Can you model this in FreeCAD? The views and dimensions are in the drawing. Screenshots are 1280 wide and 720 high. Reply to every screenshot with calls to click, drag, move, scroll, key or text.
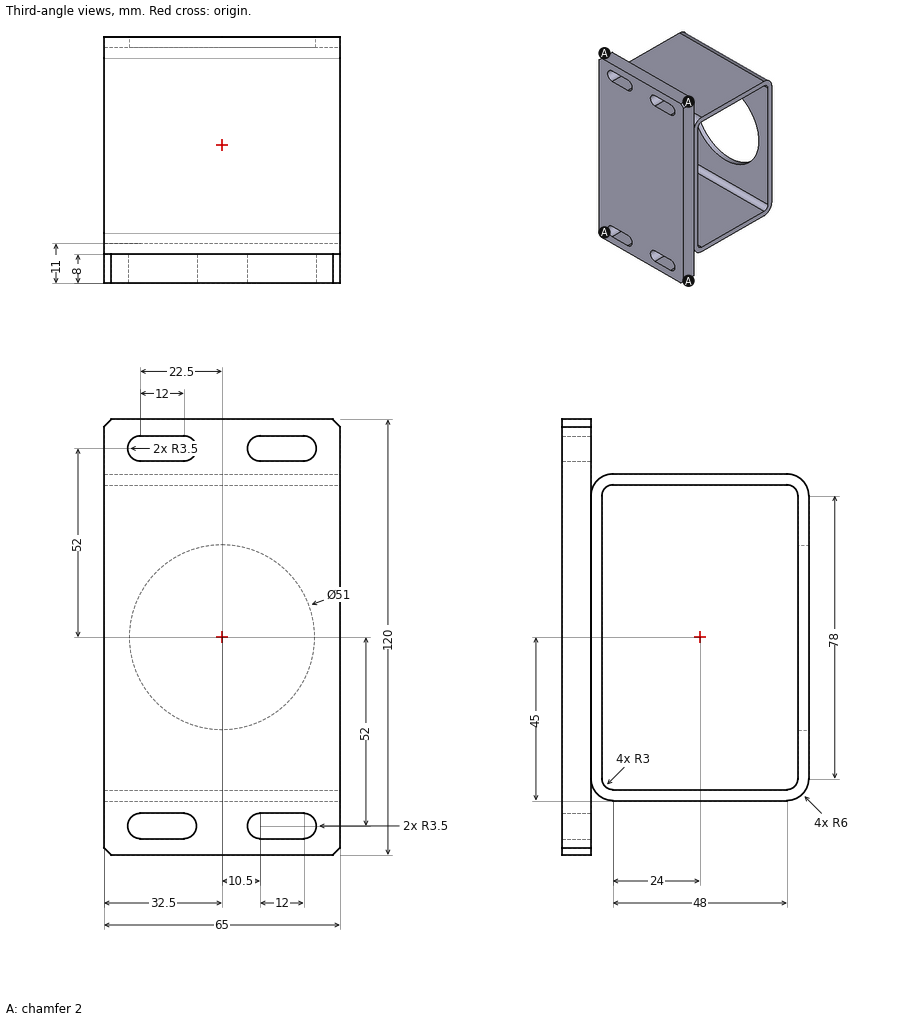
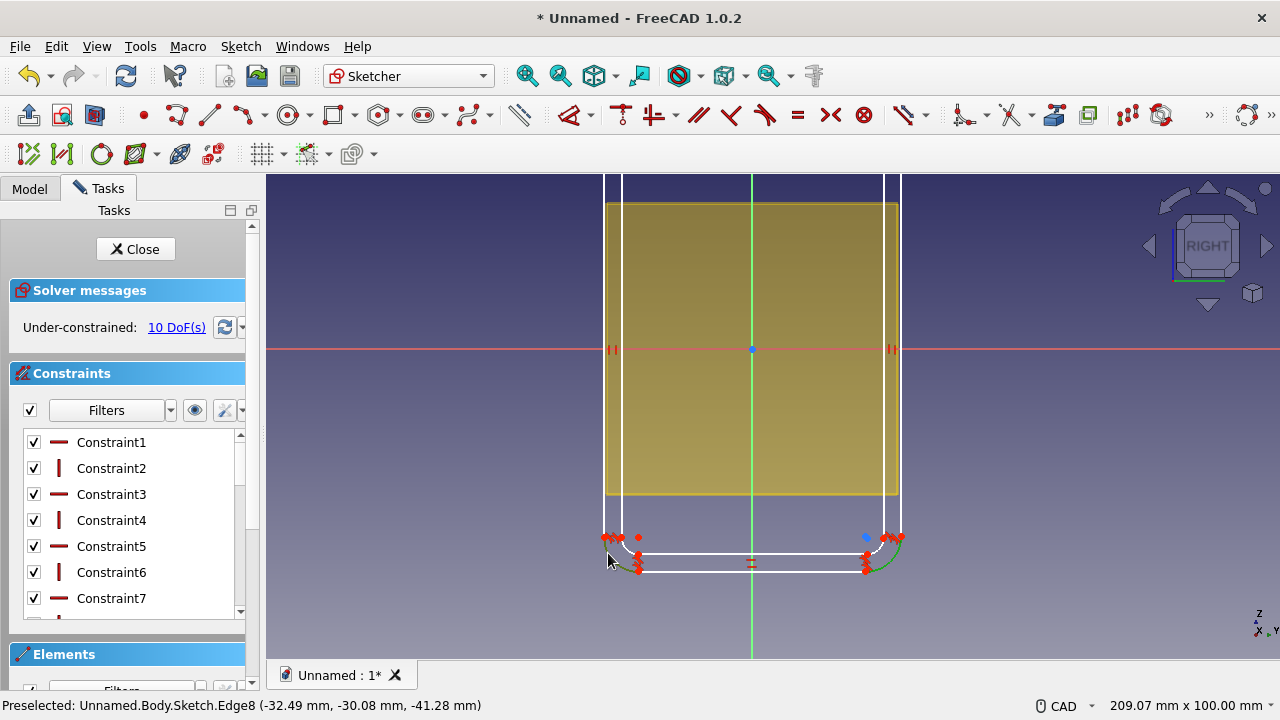
click(798, 116)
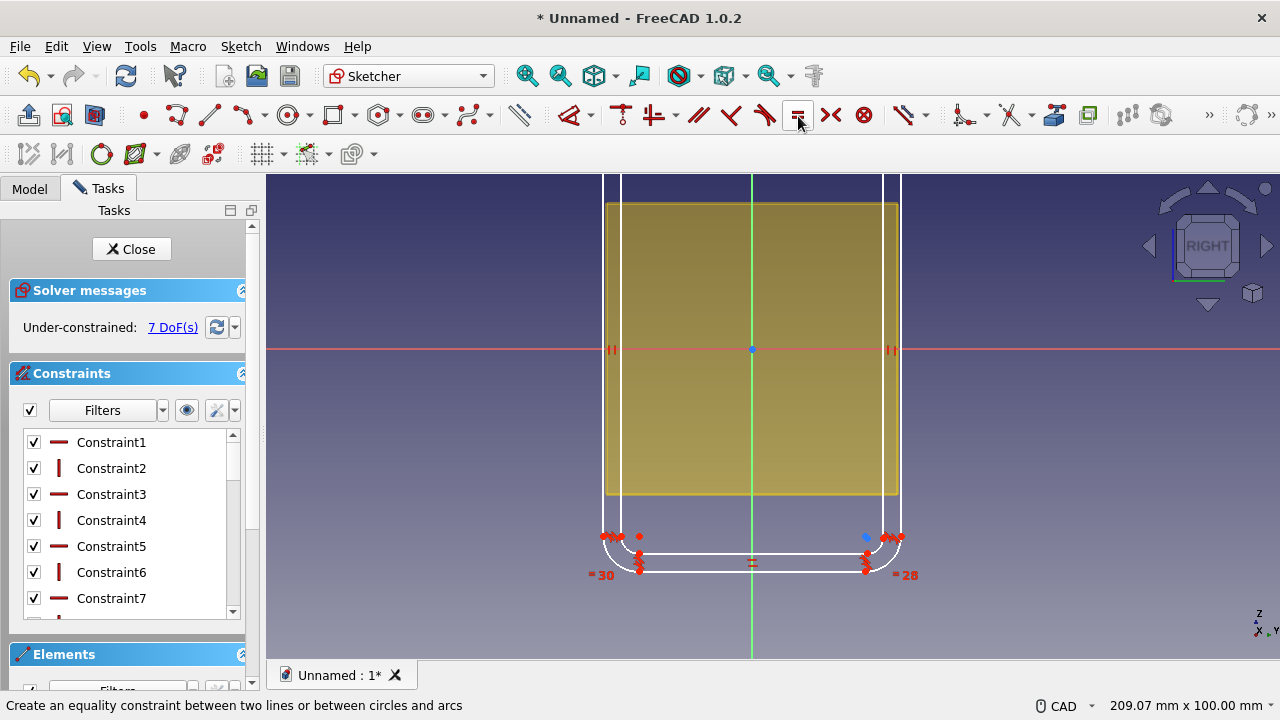
click(626, 549)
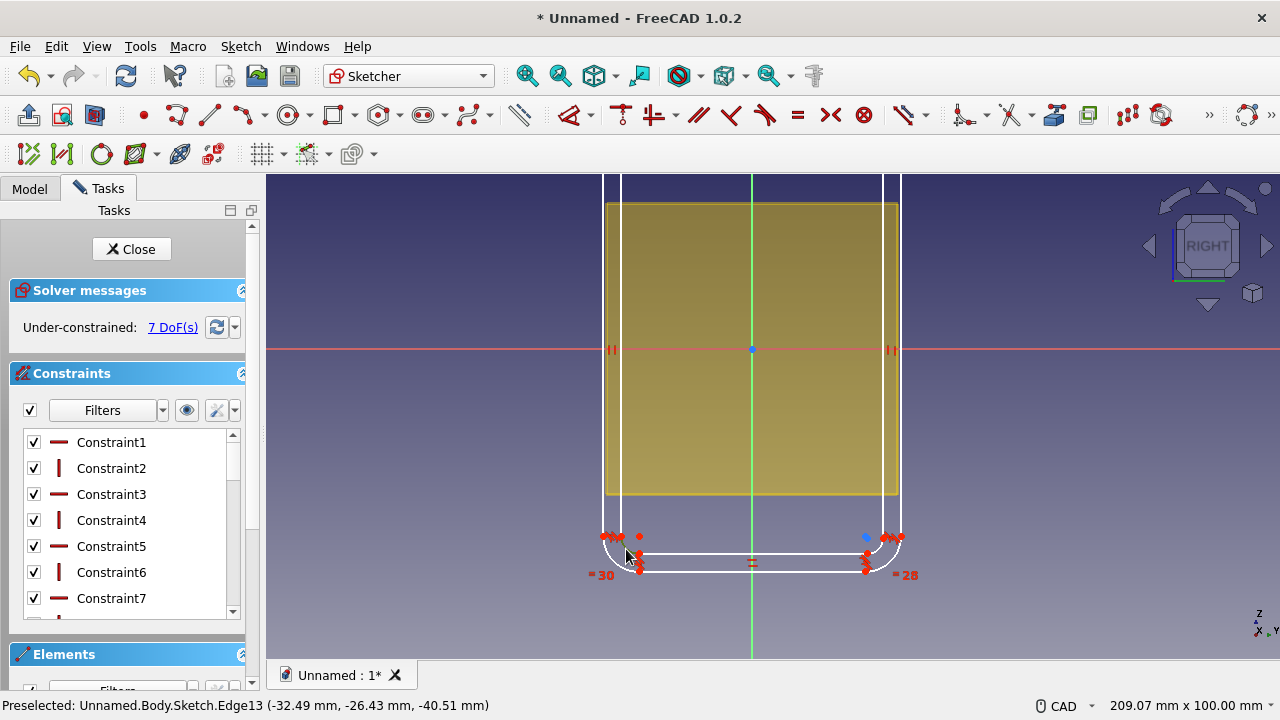
click(878, 549)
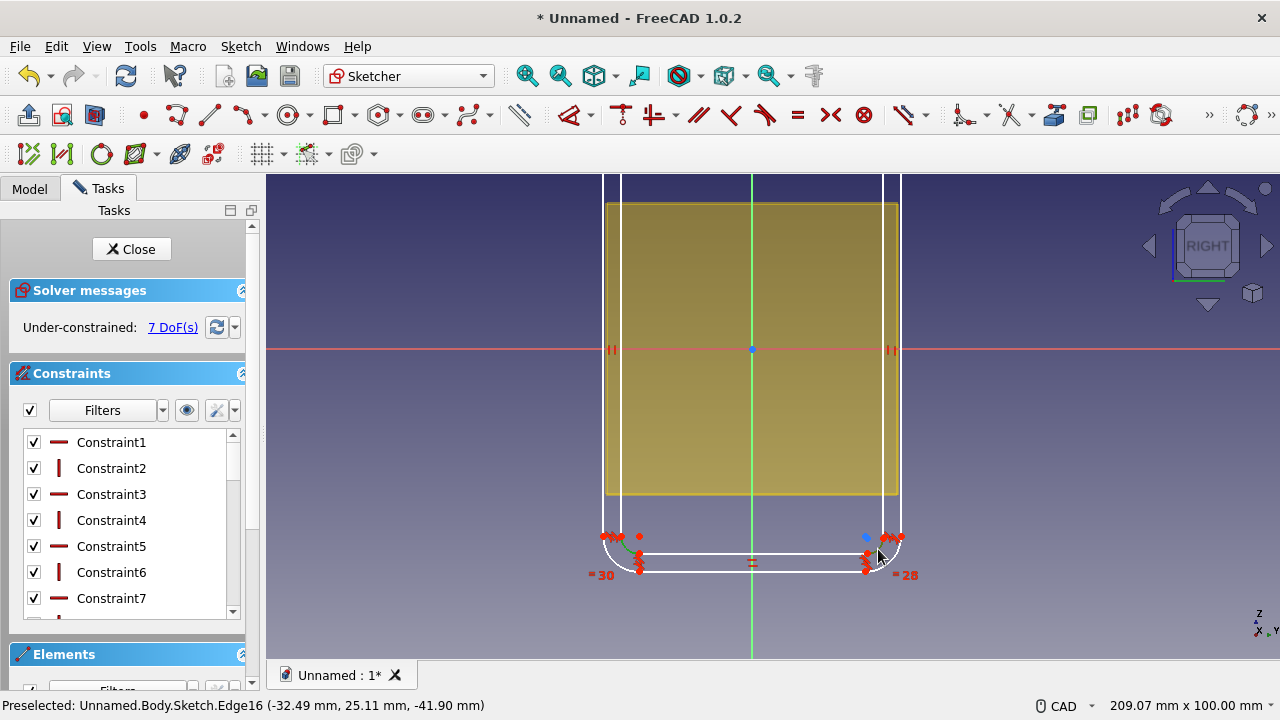
click(798, 116)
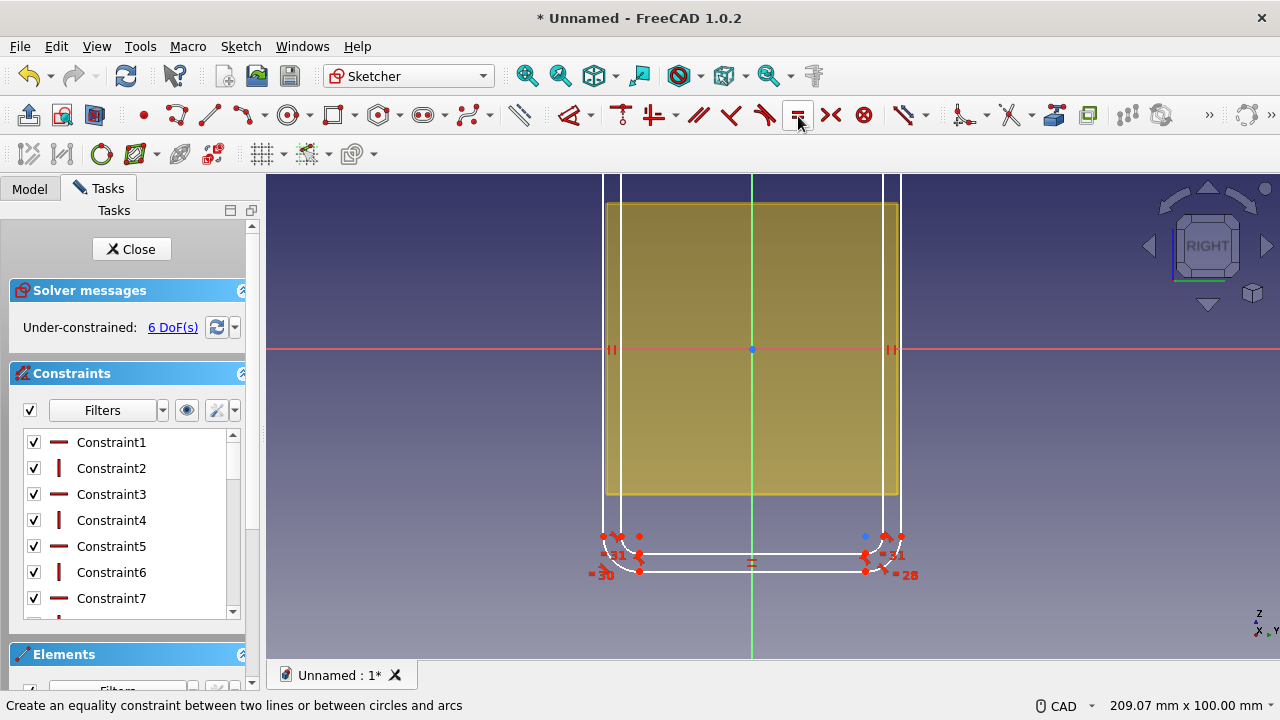
click(568, 116)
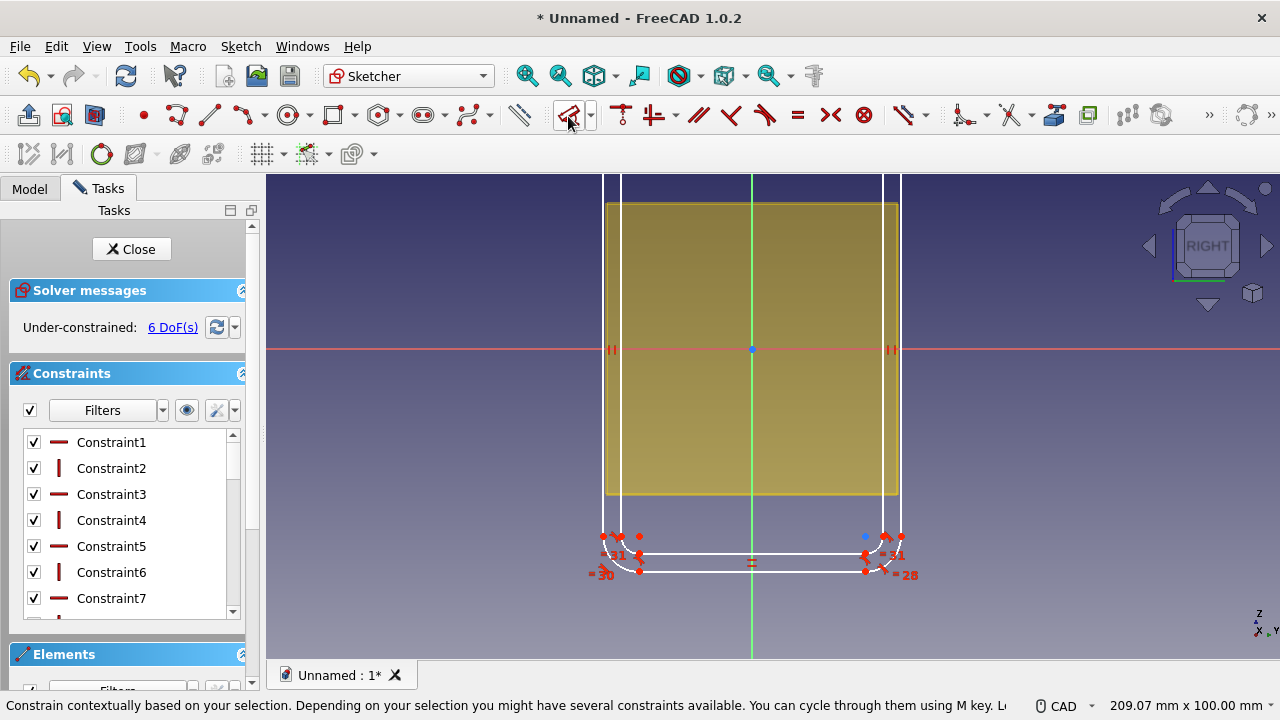
scroll(882, 568, up, 2)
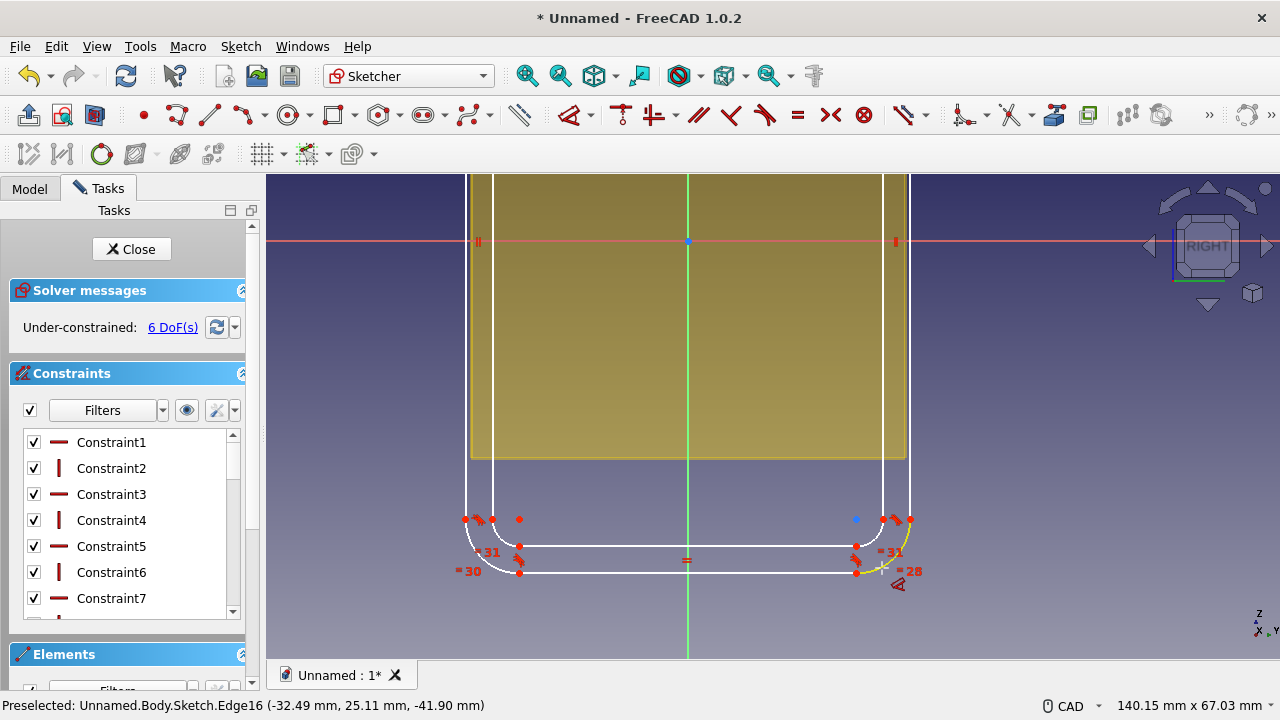
click(881, 568)
click(895, 597)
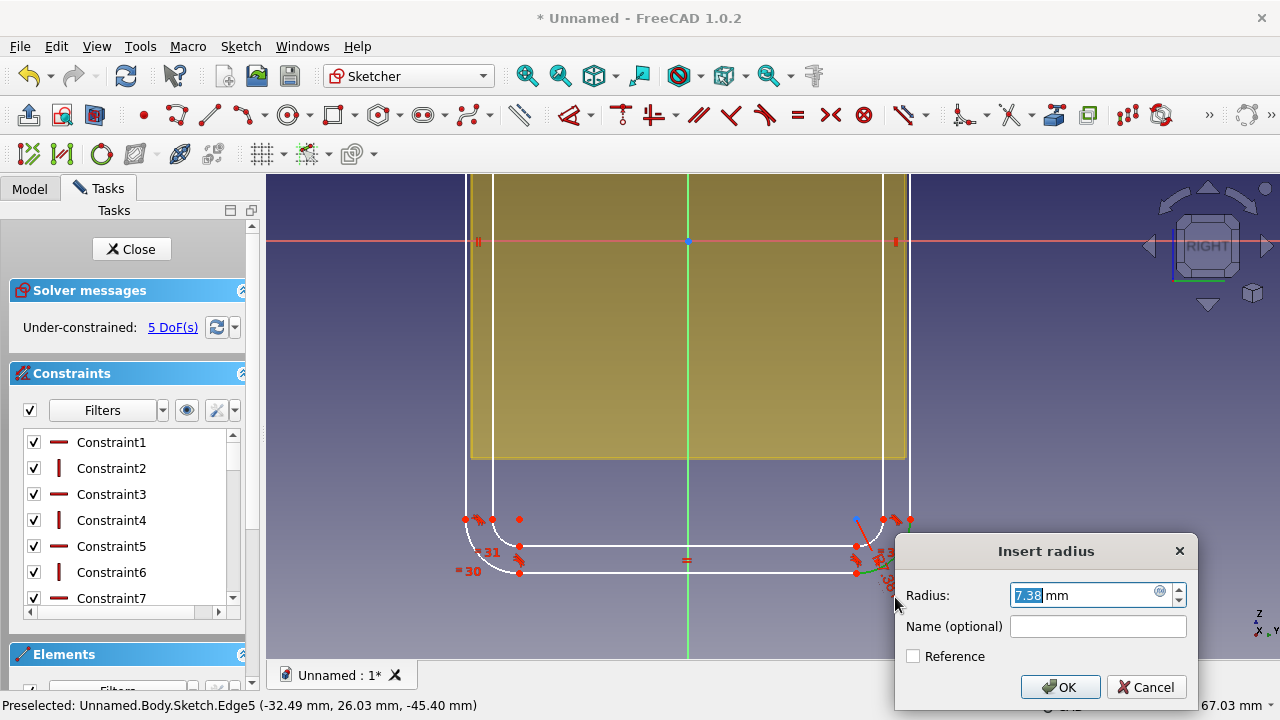
text(6)
key(Return)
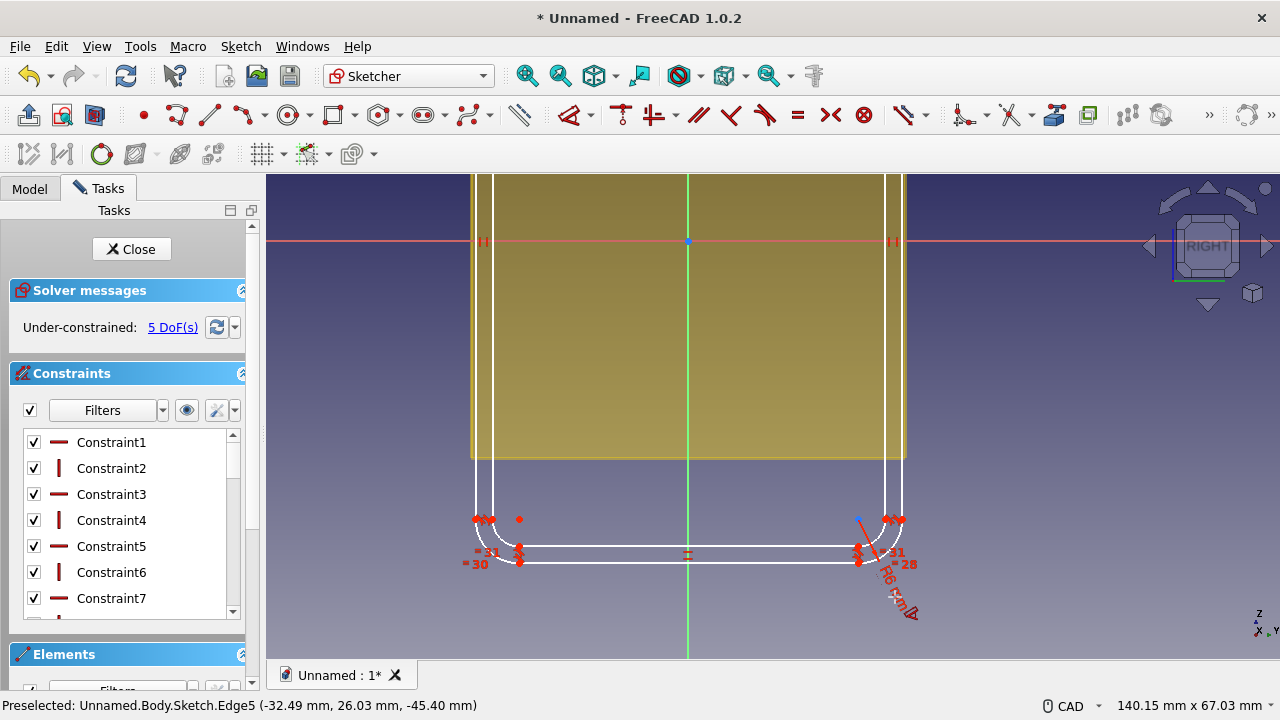
scroll(496, 532, up, 4)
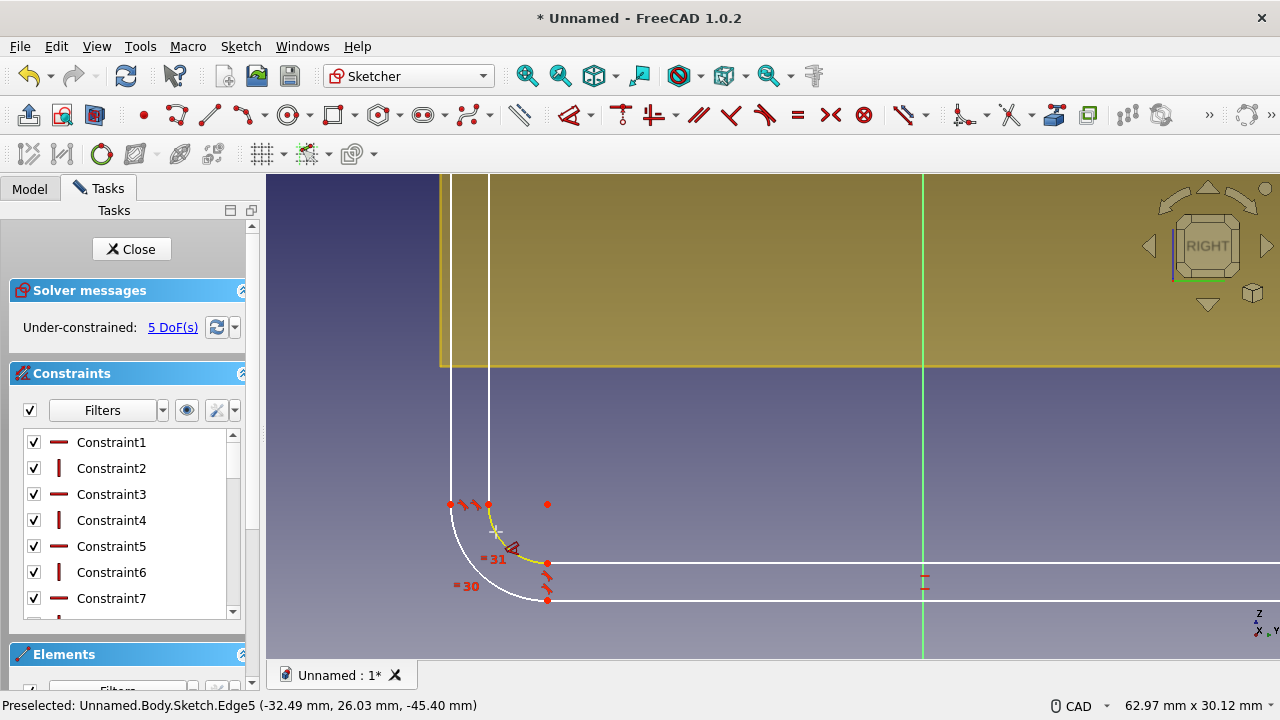
click(495, 531)
click(469, 458)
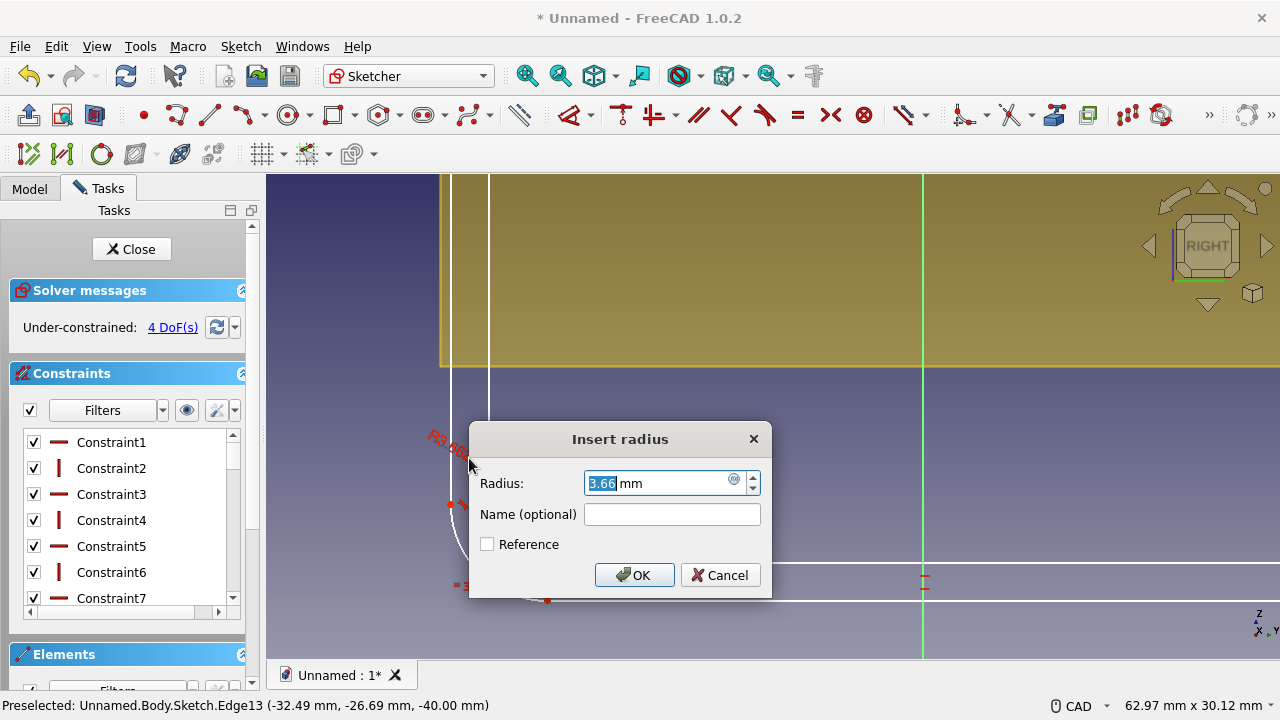
text(3)
key(Return)